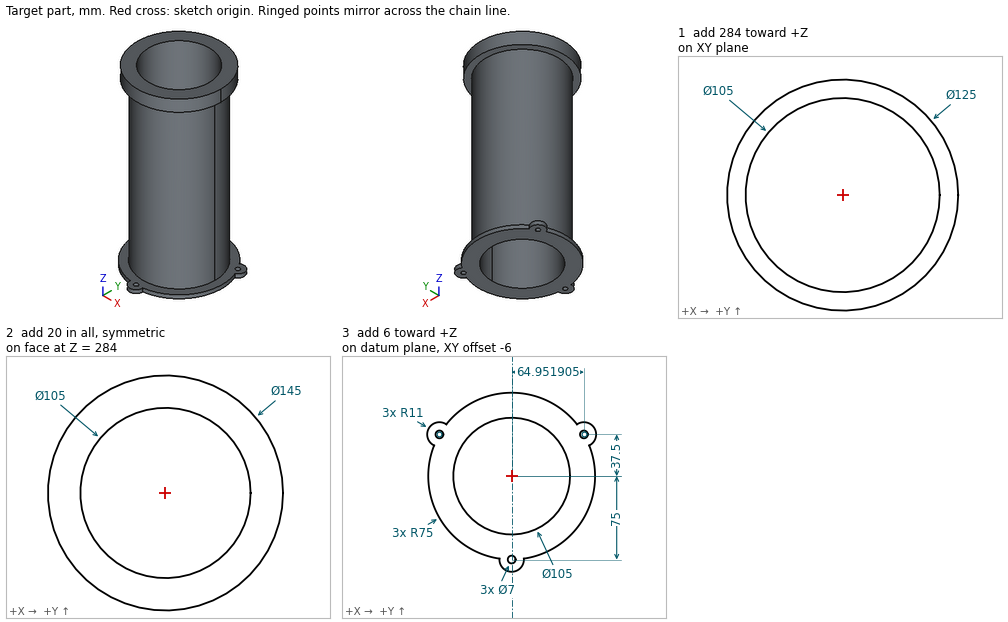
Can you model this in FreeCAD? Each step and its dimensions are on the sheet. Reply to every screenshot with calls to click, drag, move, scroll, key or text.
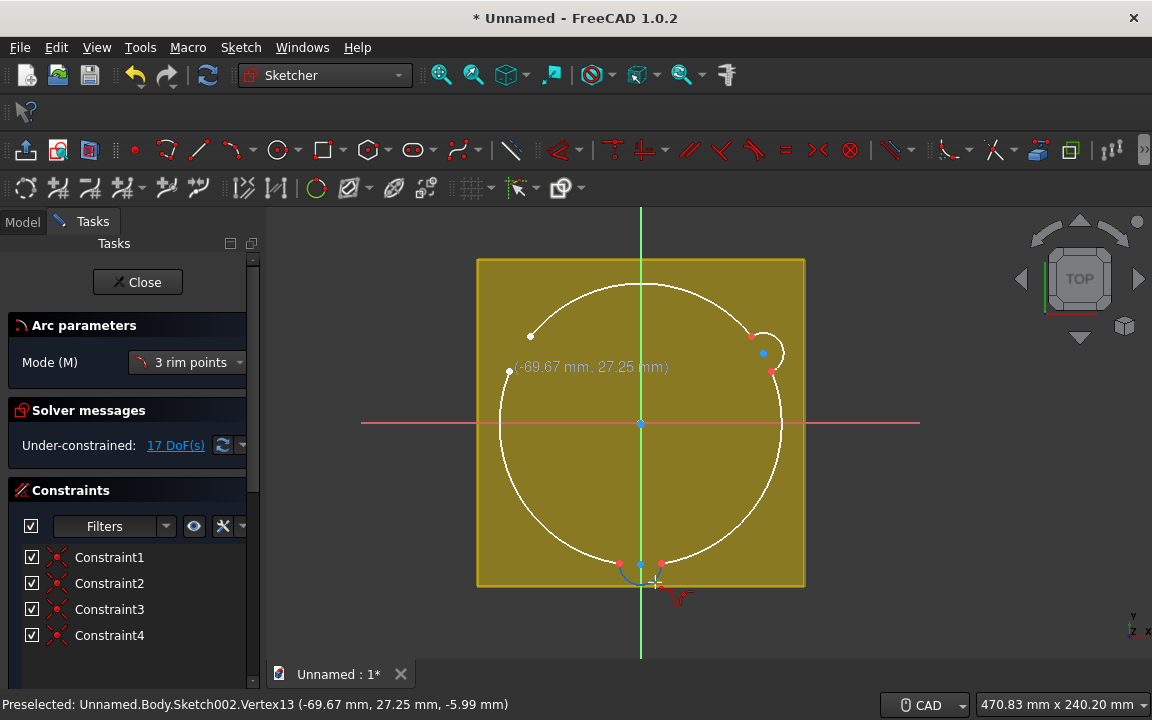
click(531, 337)
click(501, 342)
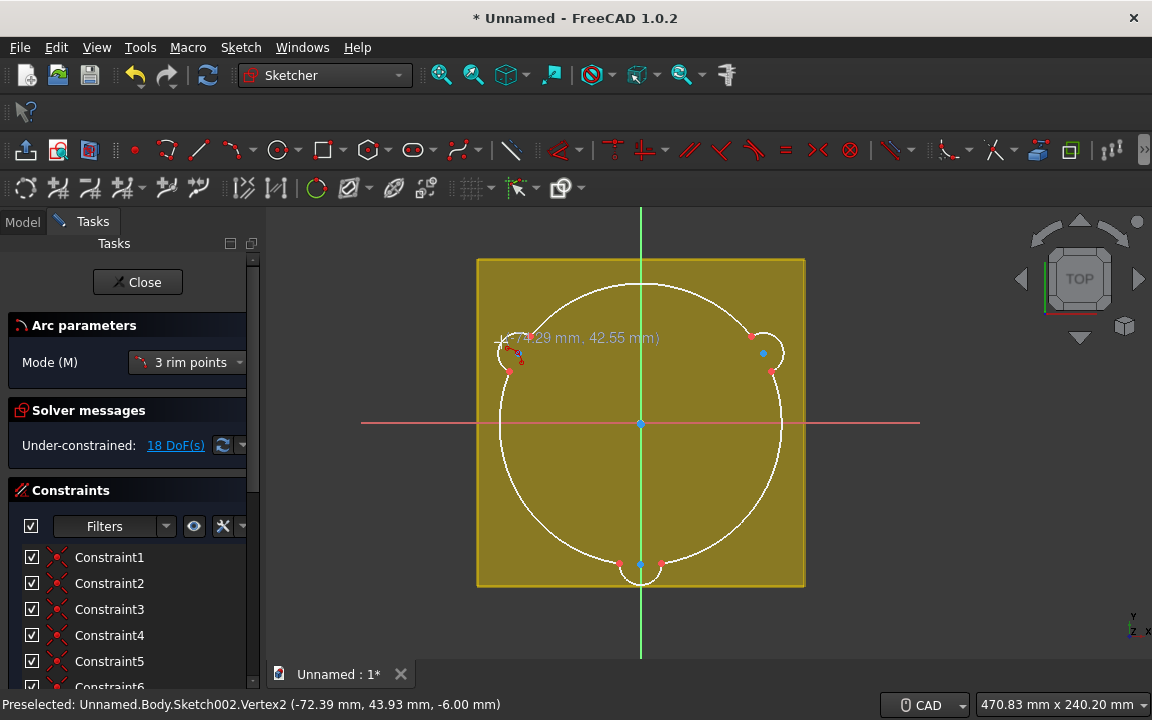
click(278, 150)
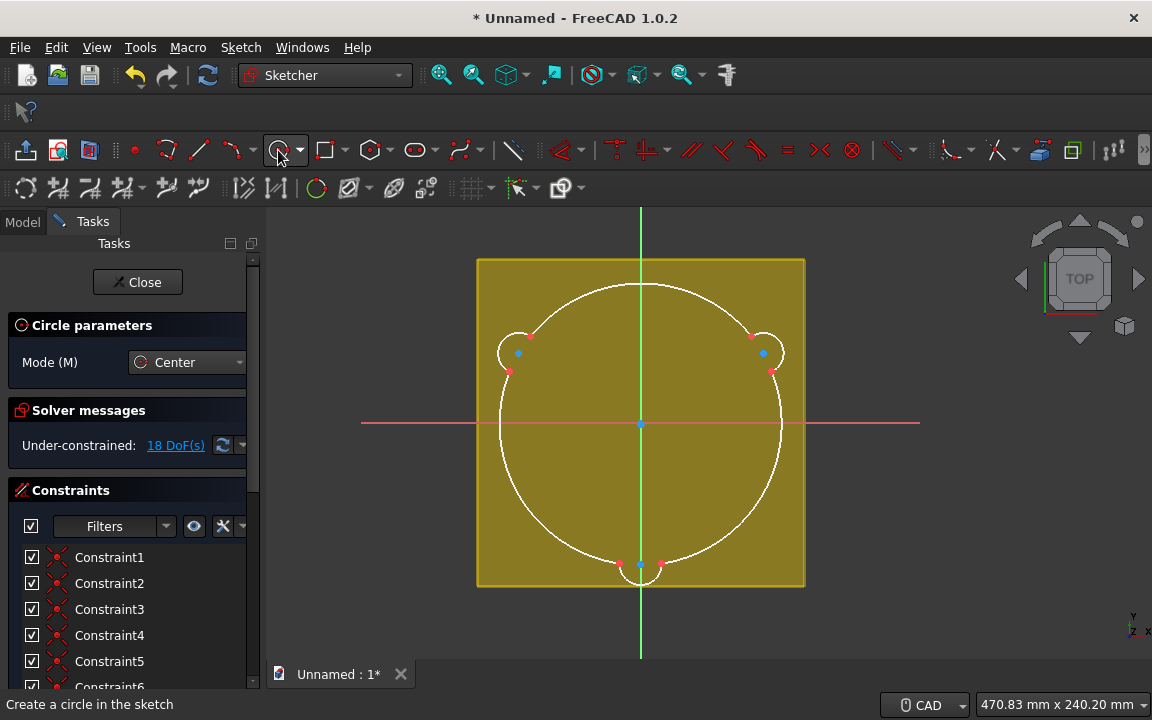
scroll(641, 564, up, 7)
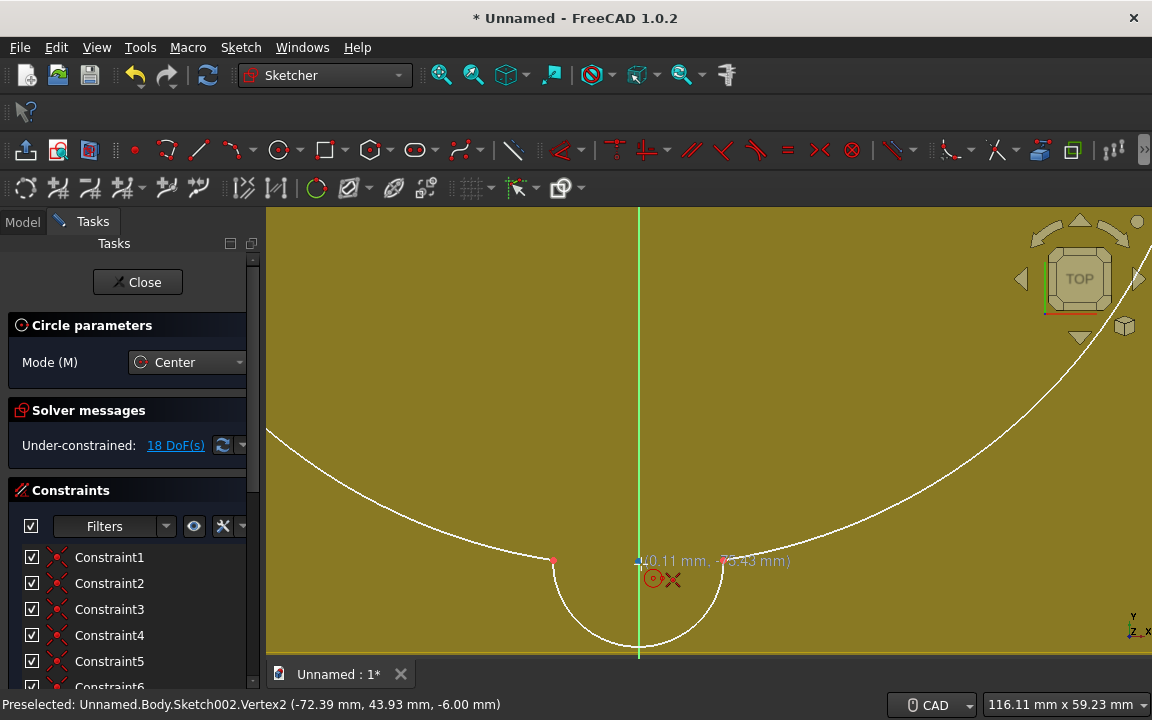
scroll(641, 564, down, 7)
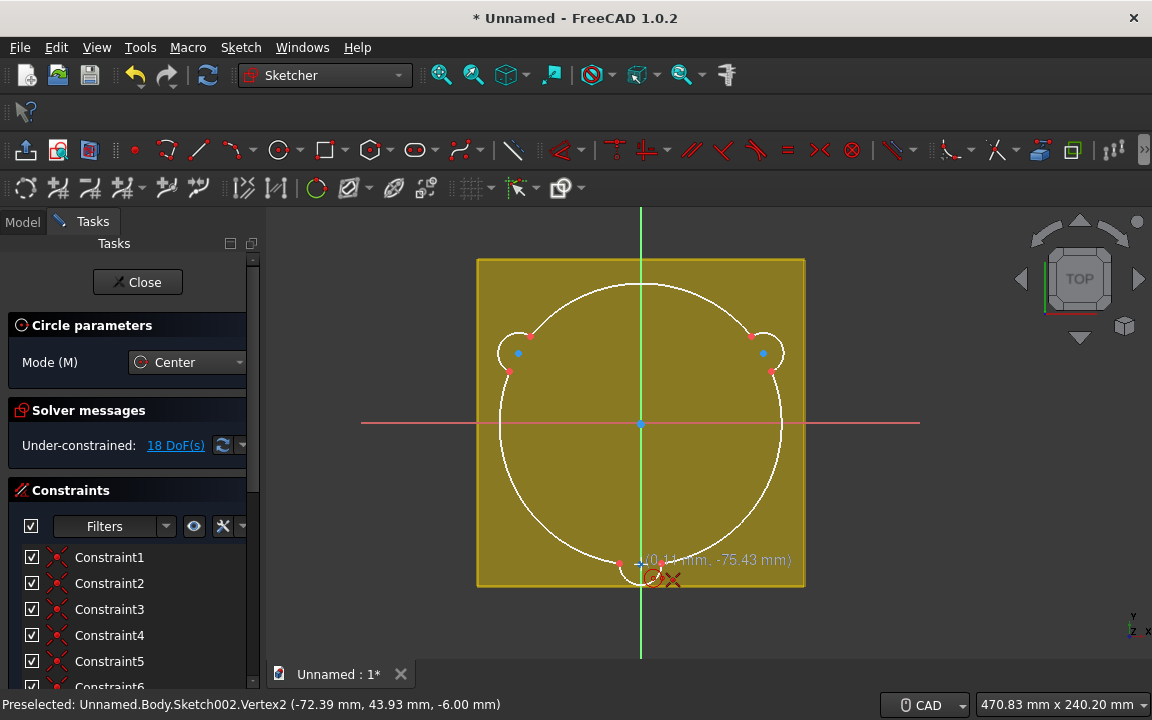
click(641, 564)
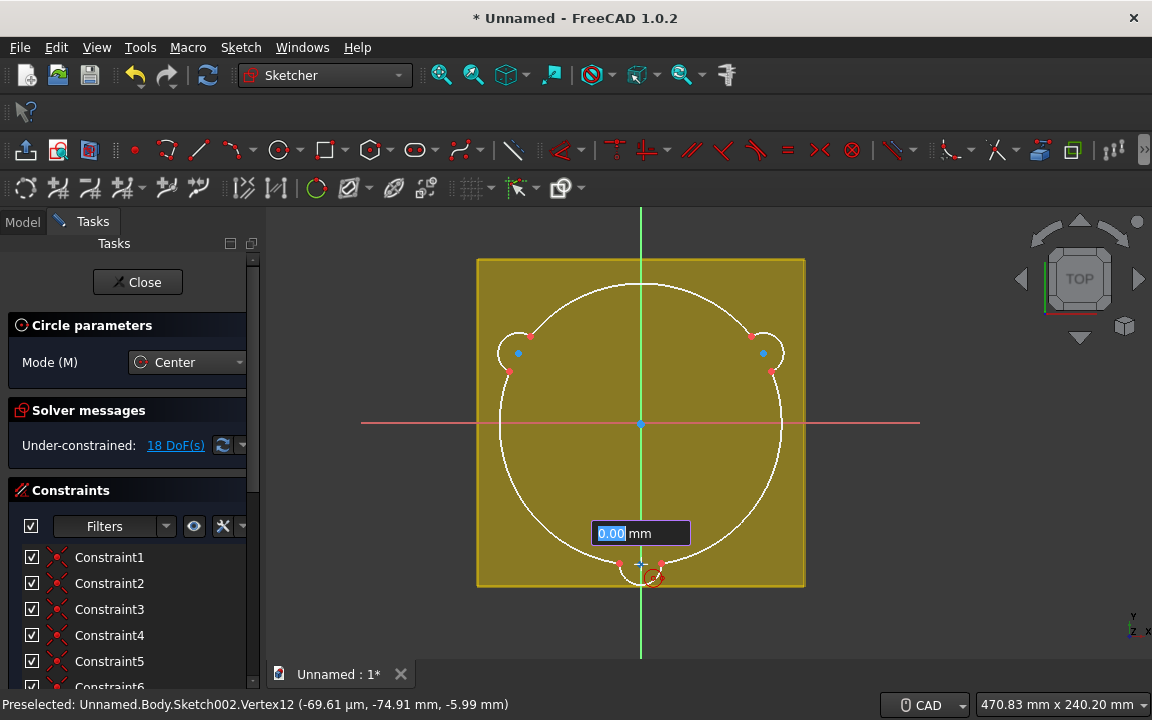
scroll(647, 562, up, 5)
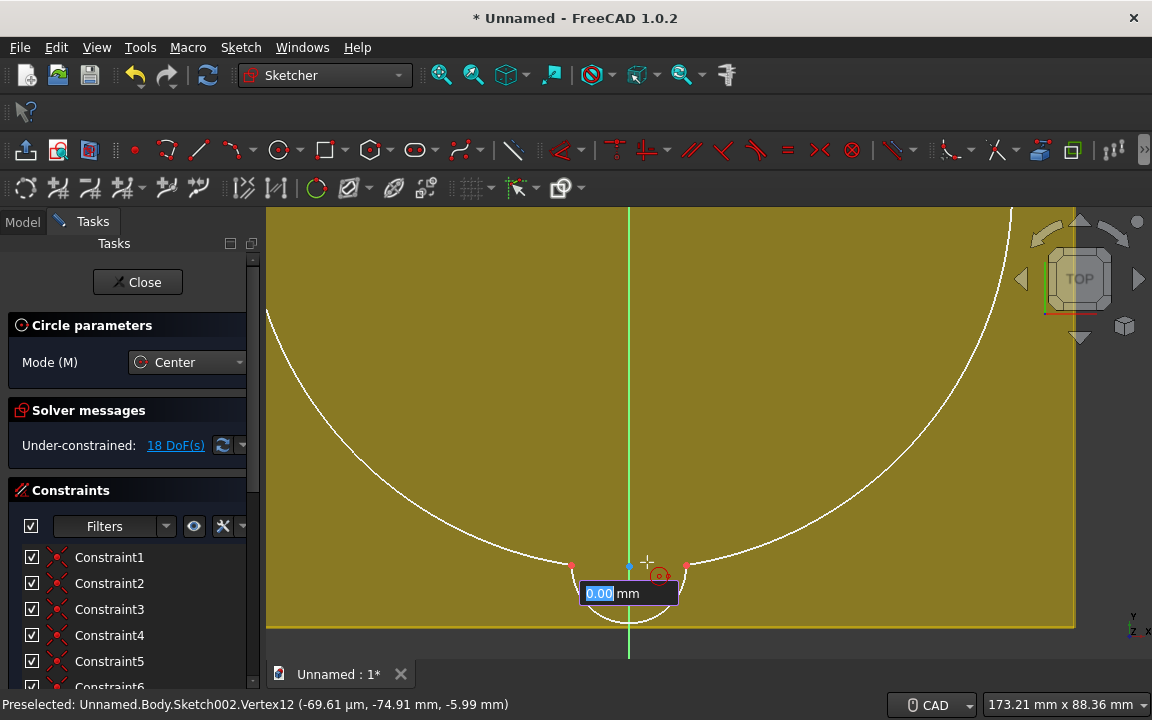
click(646, 560)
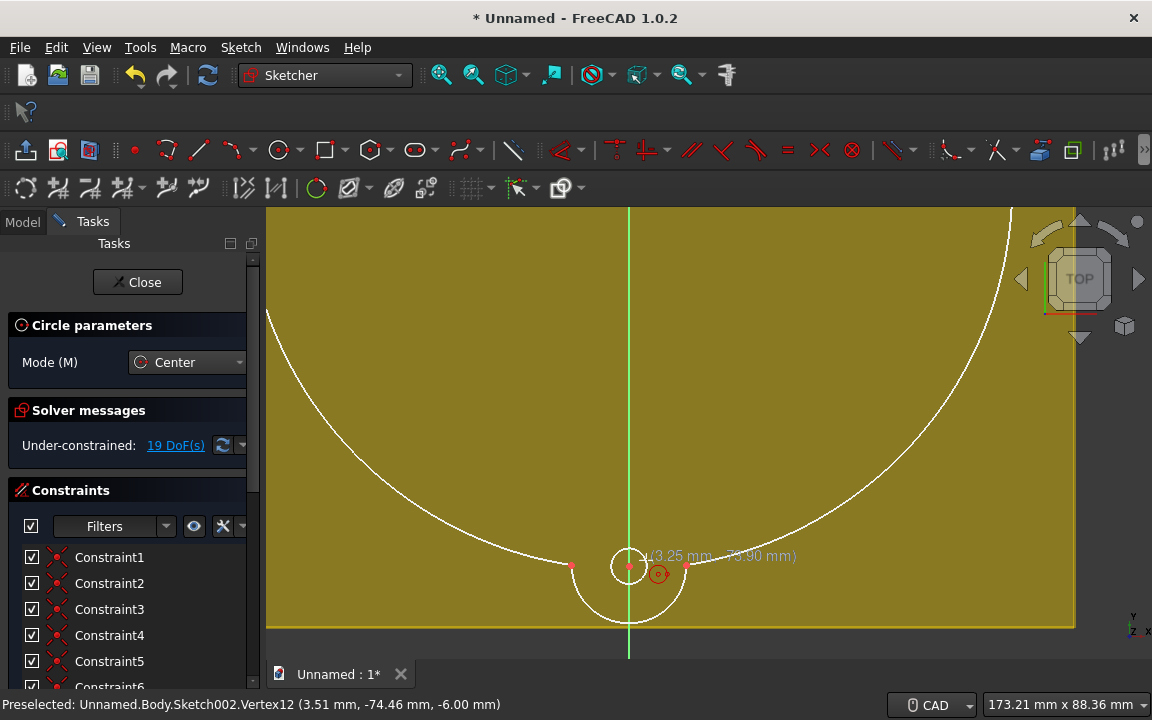
scroll(647, 562, down, 5)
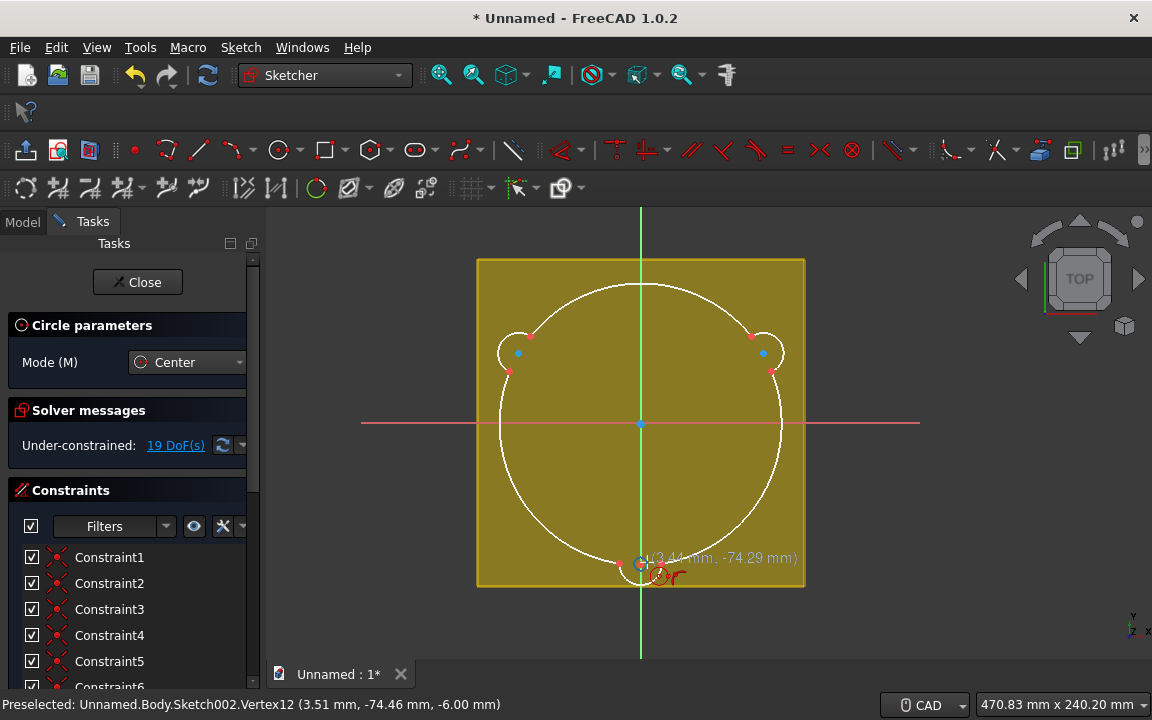
scroll(763, 352, up, 7)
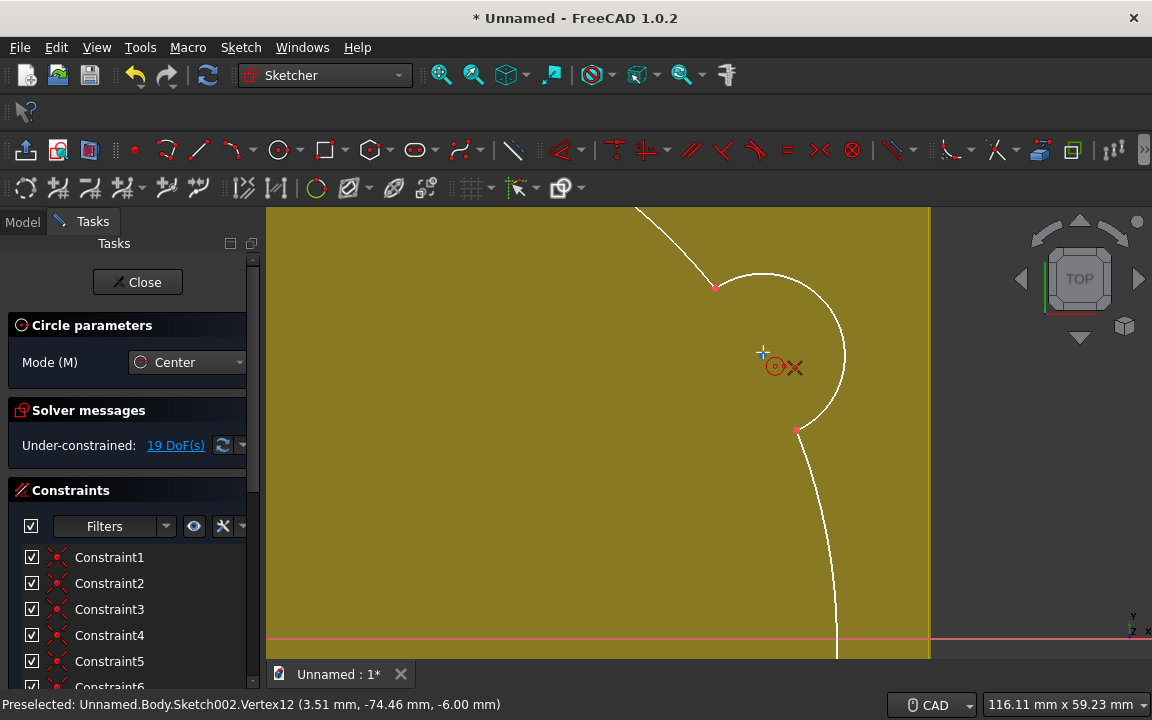
scroll(763, 352, down, 7)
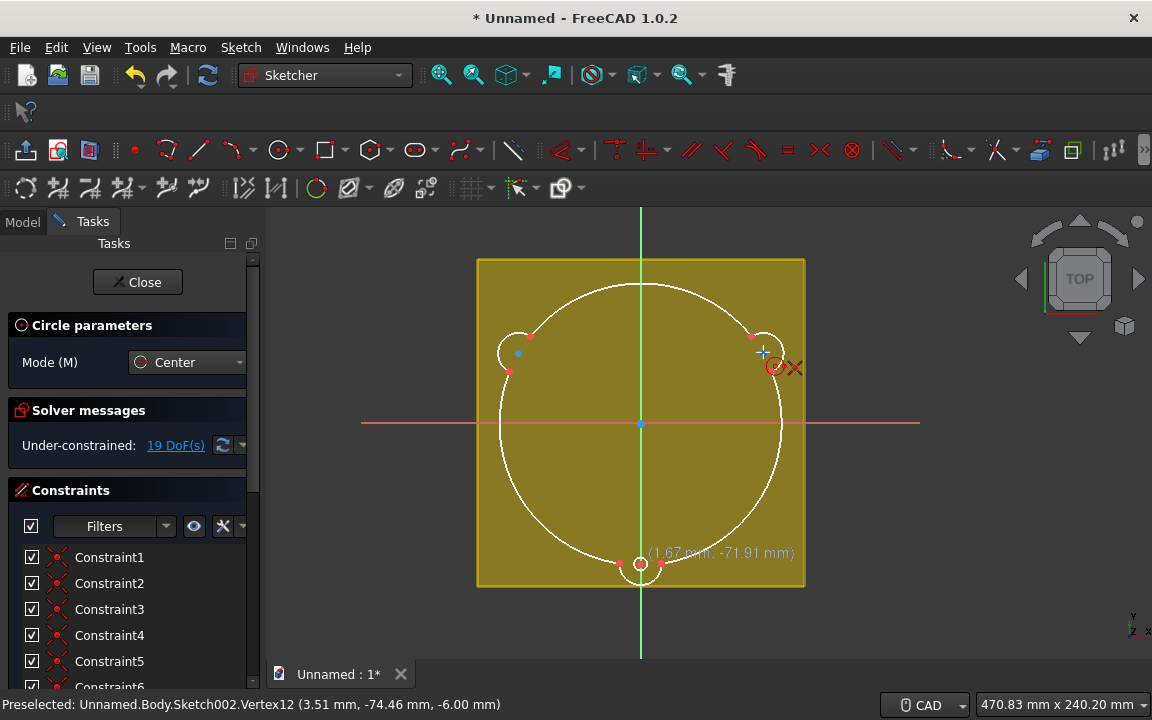
click(763, 352)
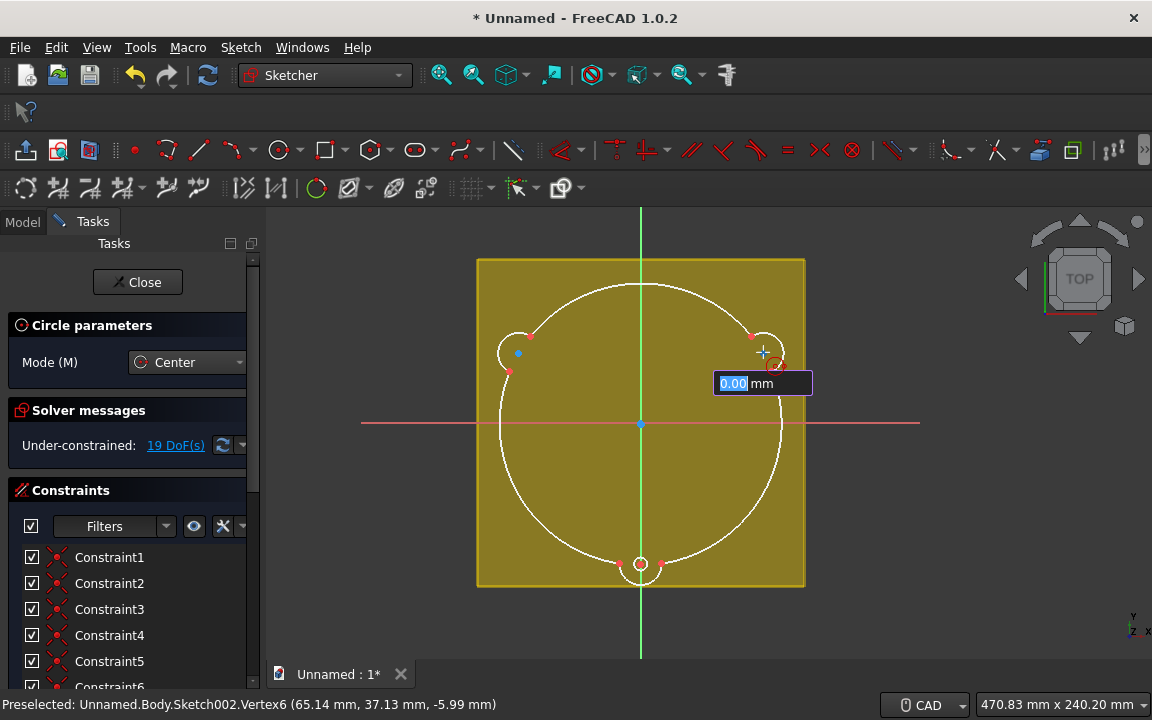
scroll(769, 350, up, 5)